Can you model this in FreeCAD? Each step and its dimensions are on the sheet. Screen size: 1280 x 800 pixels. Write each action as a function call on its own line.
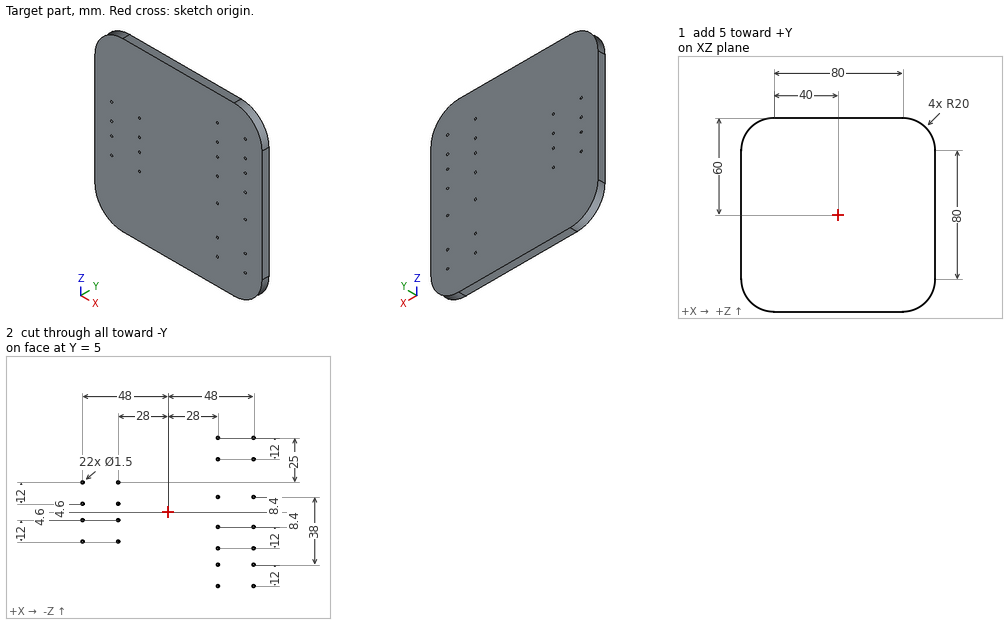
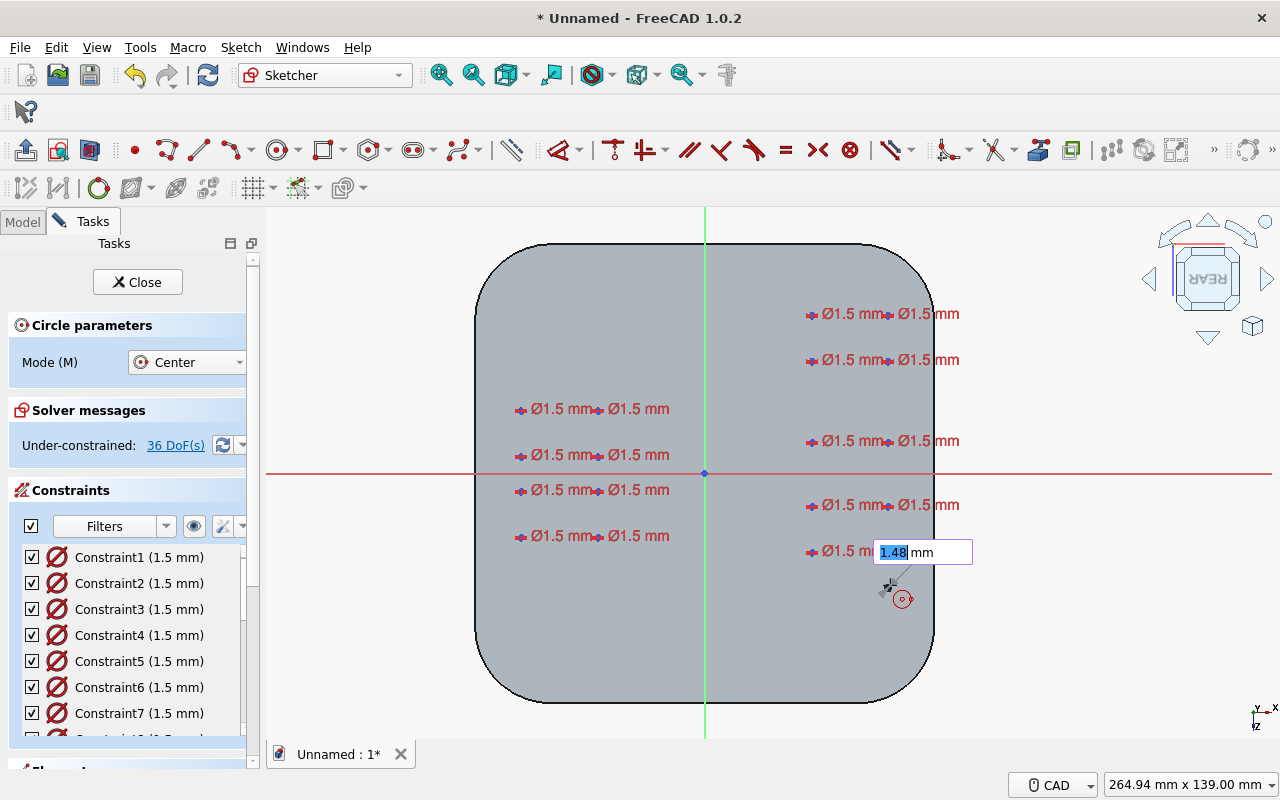
text(1.5)
key(Return)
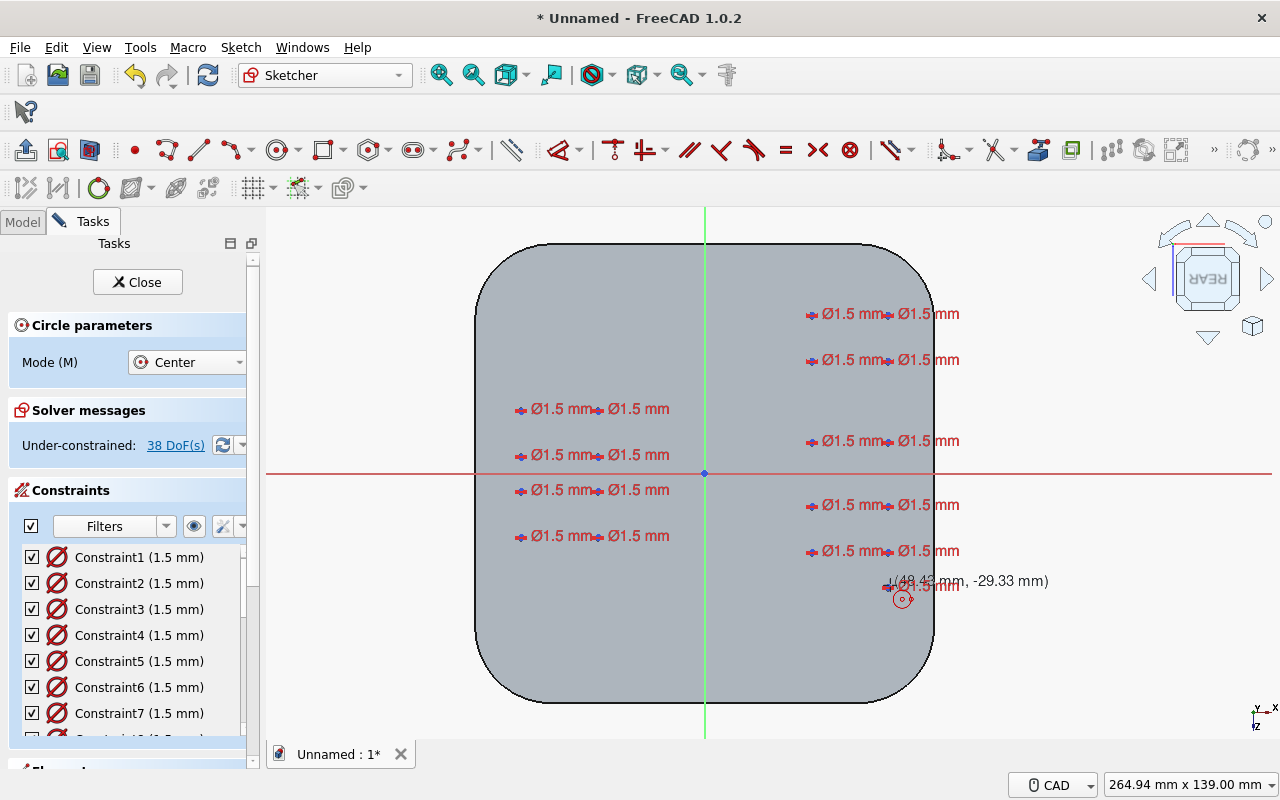
scroll(812, 587, up, 11)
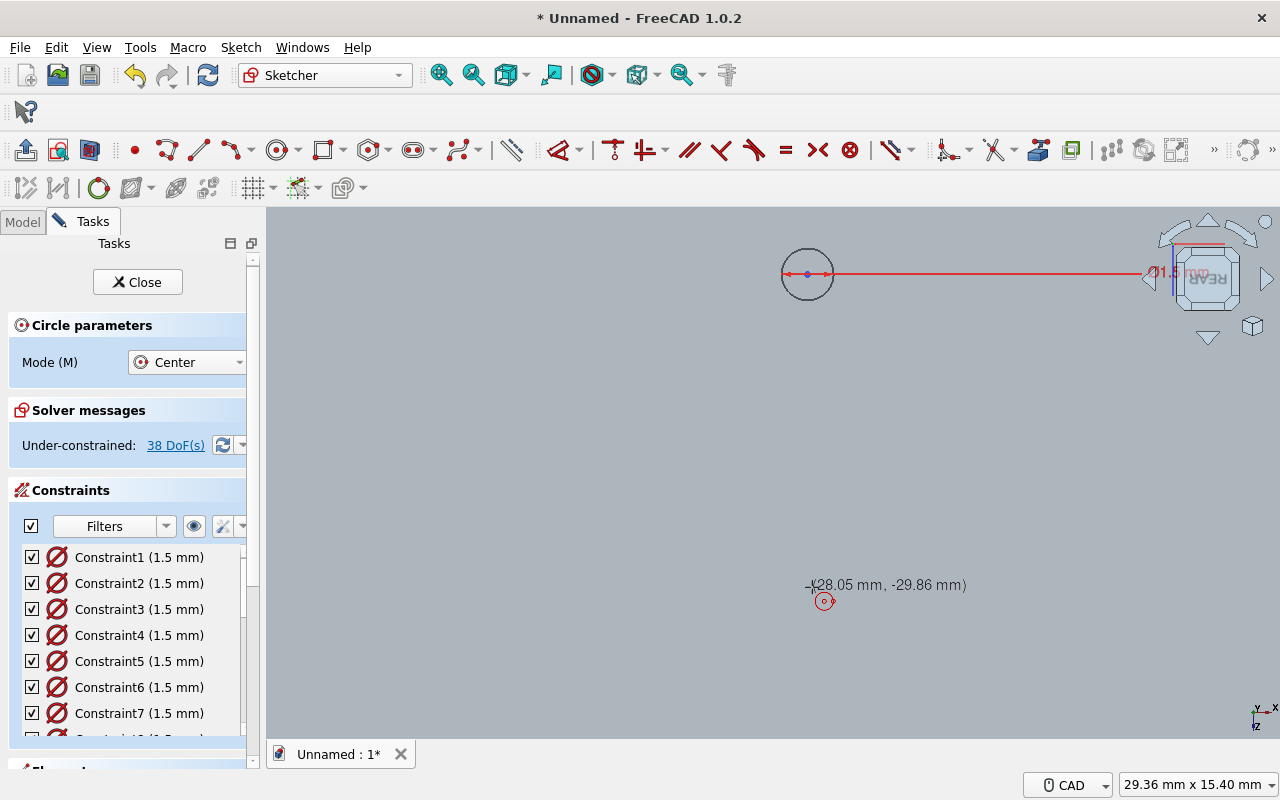
scroll(812, 587, down, 11)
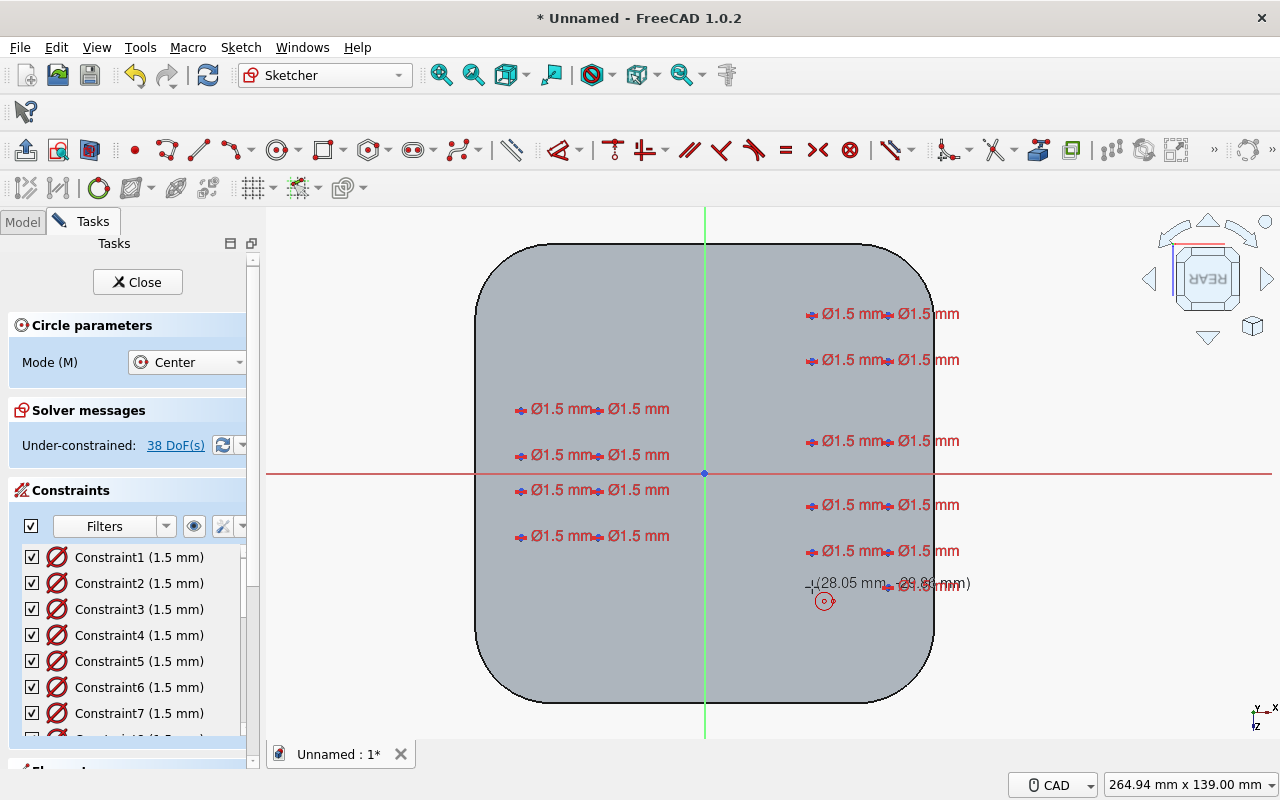
click(812, 587)
move(814, 585)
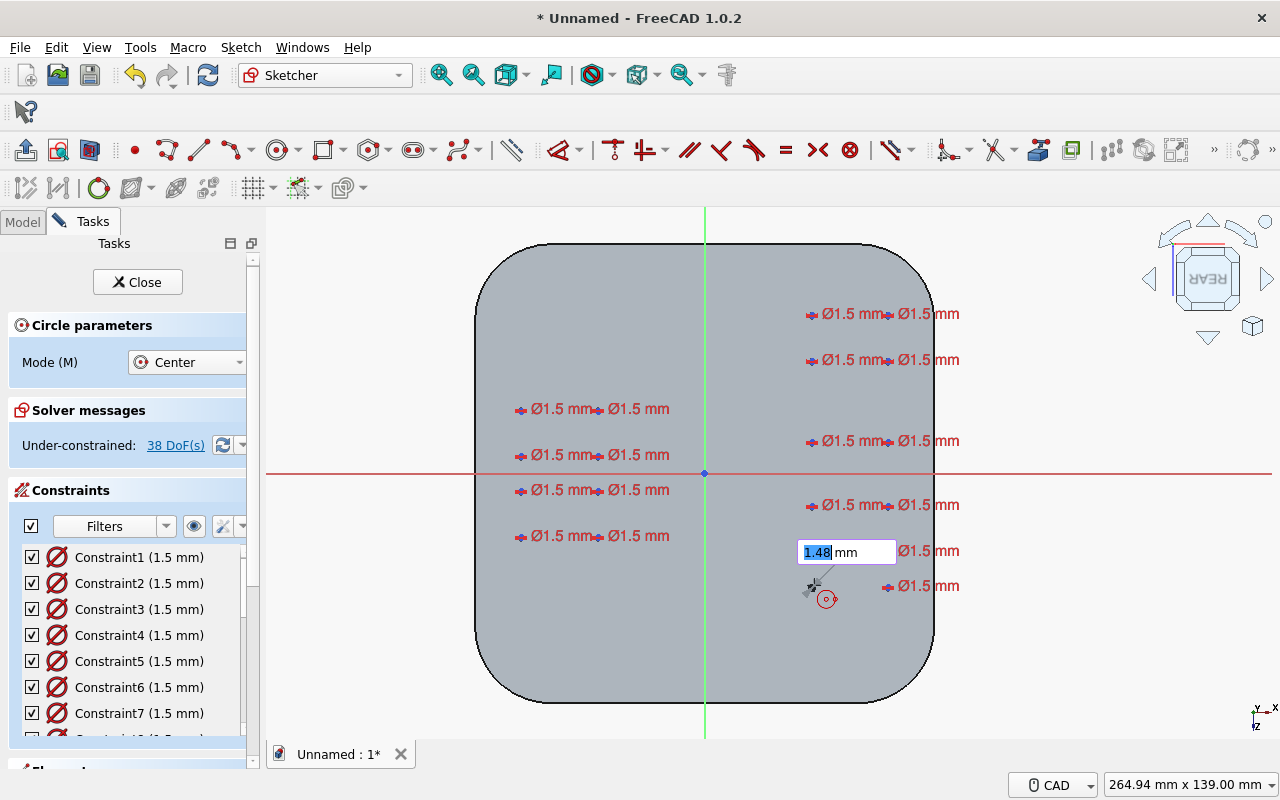
text(1.5)
key(Return)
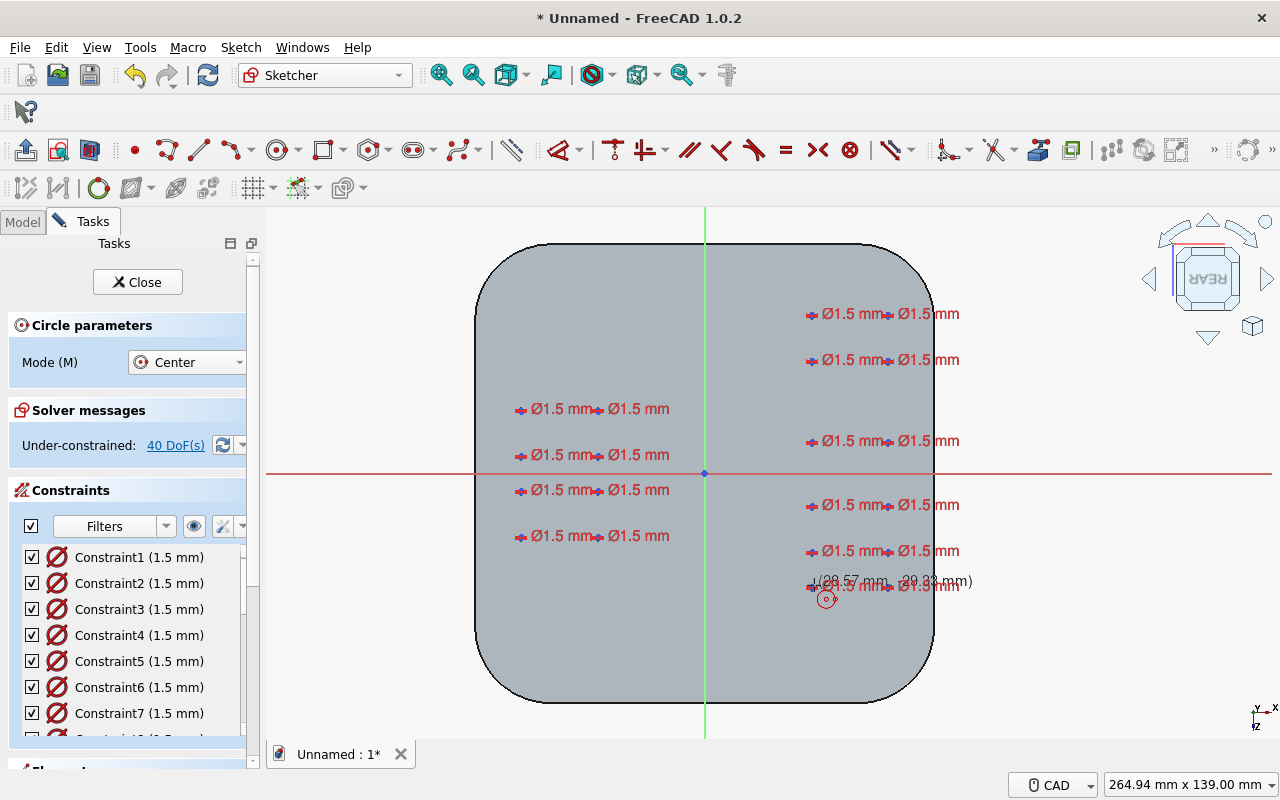
scroll(888, 633, up, 11)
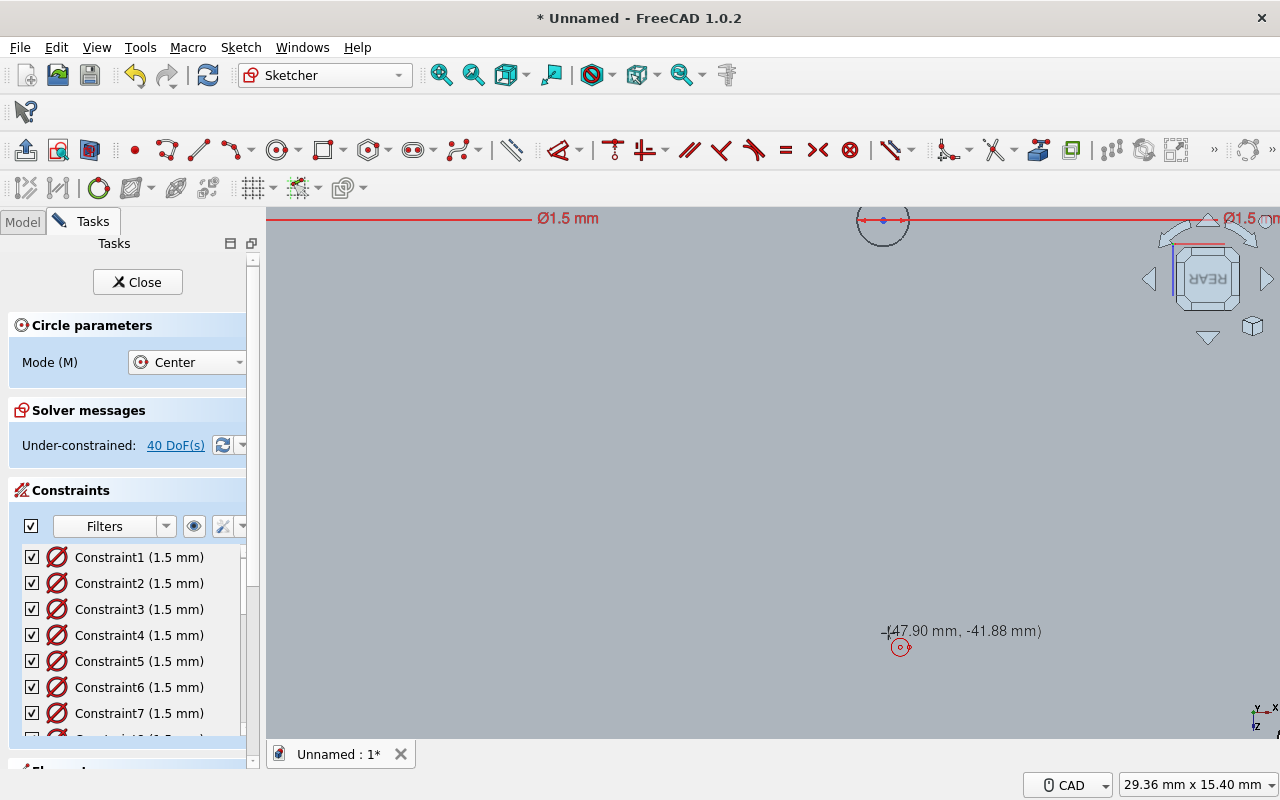
scroll(888, 633, down, 11)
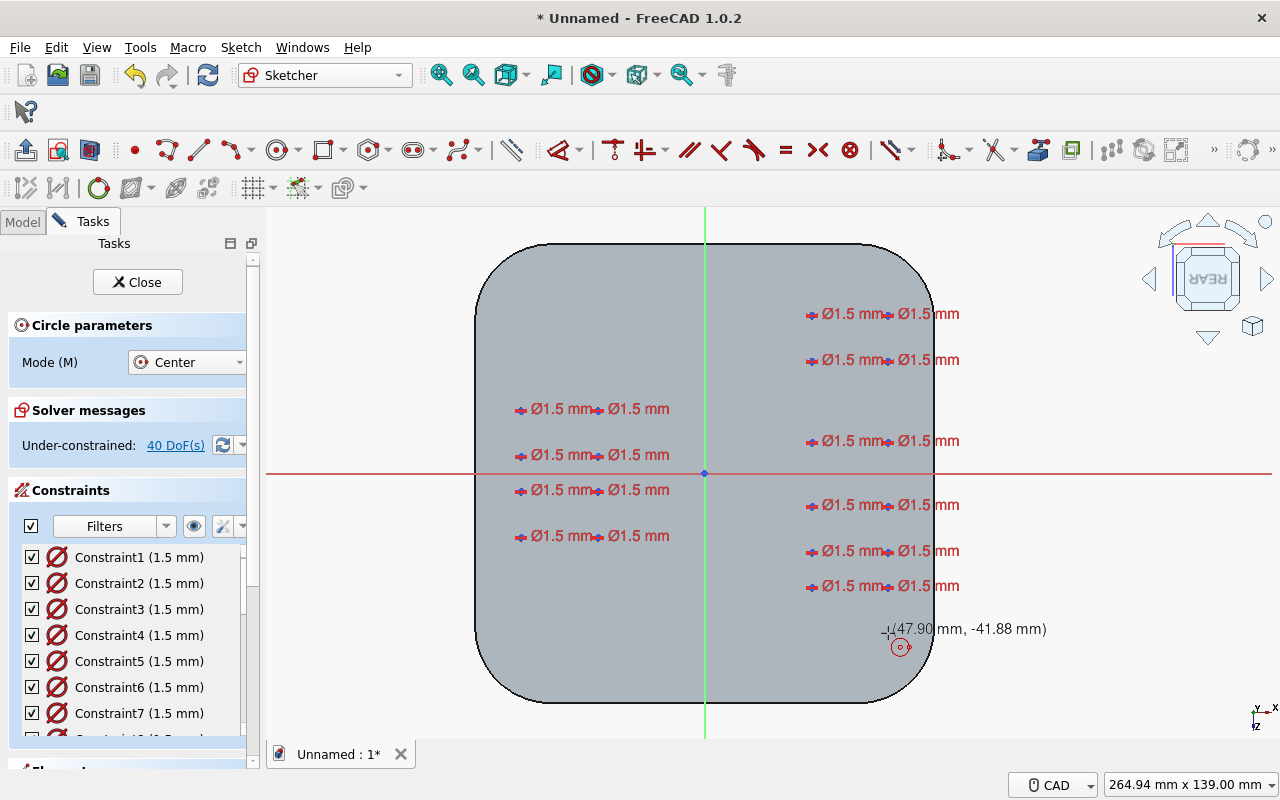
click(888, 633)
move(890, 631)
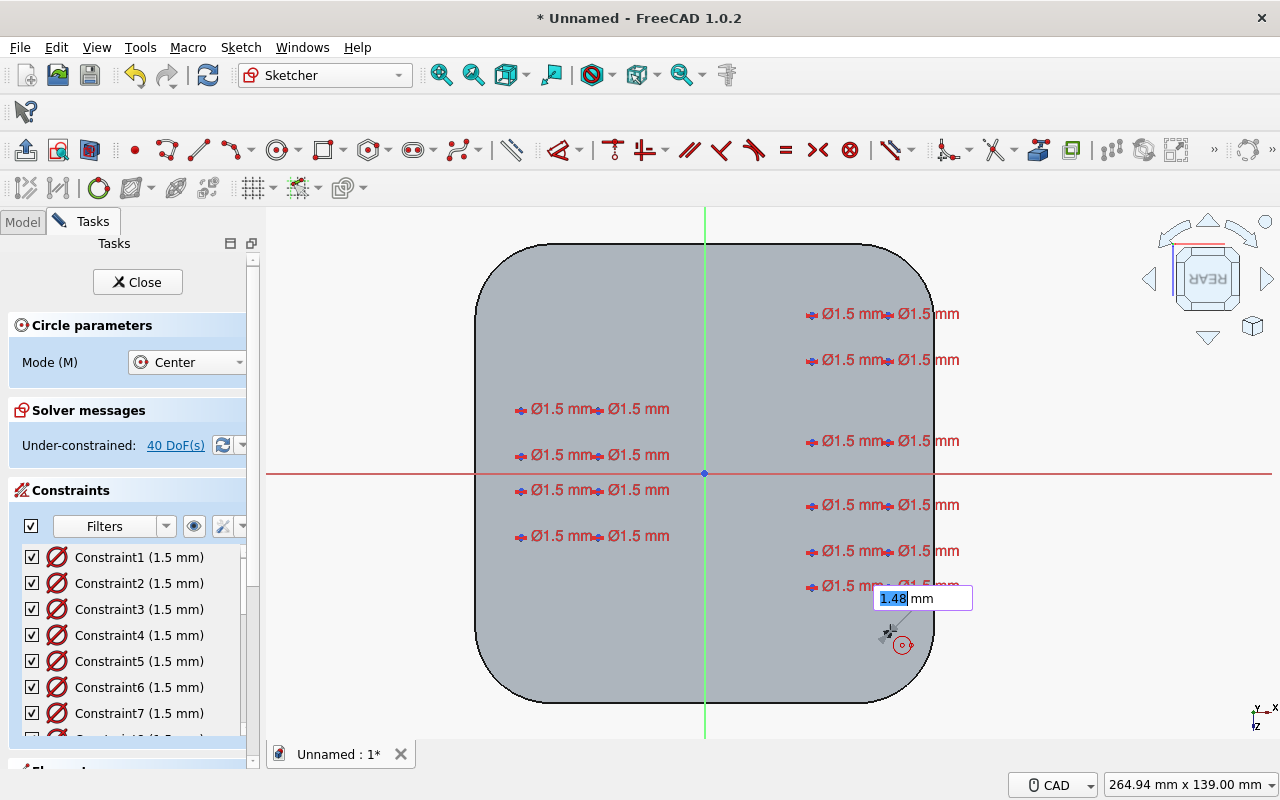
text(1.5)
key(Return)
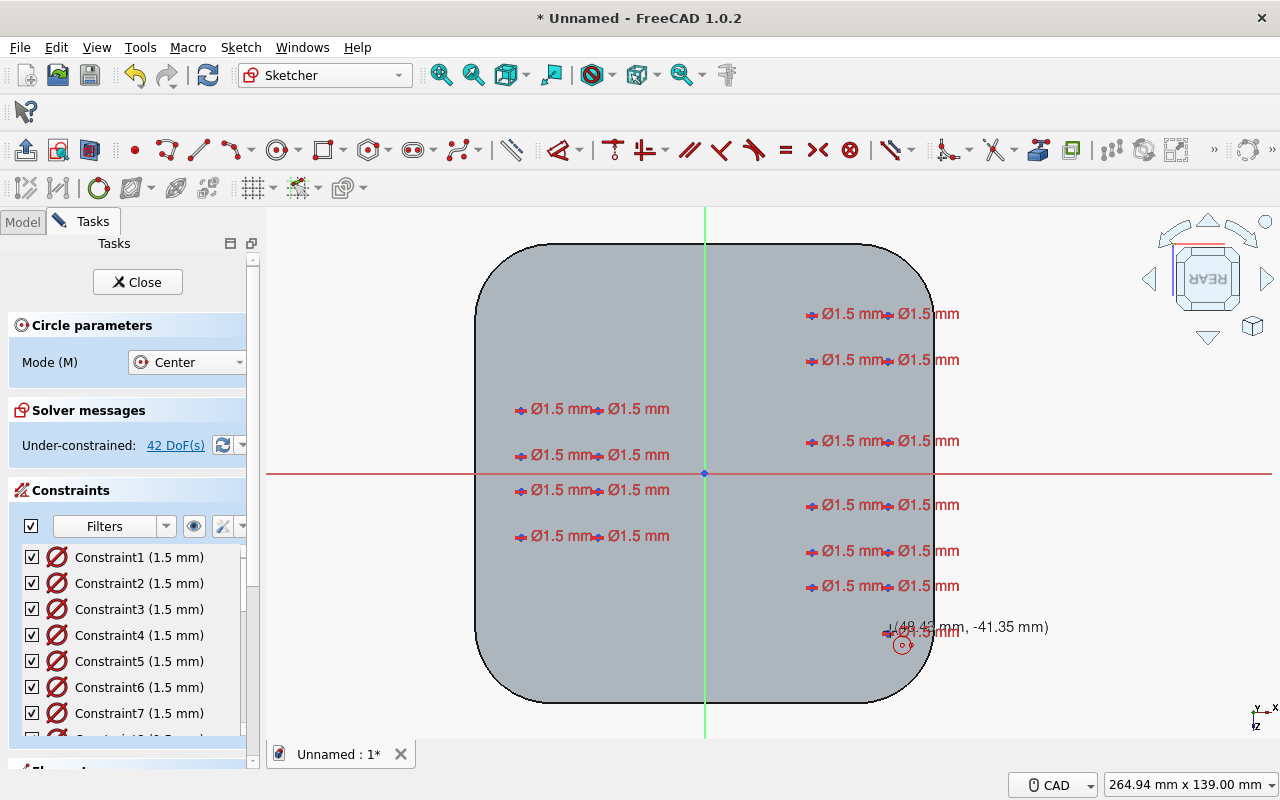
scroll(812, 633, up, 11)